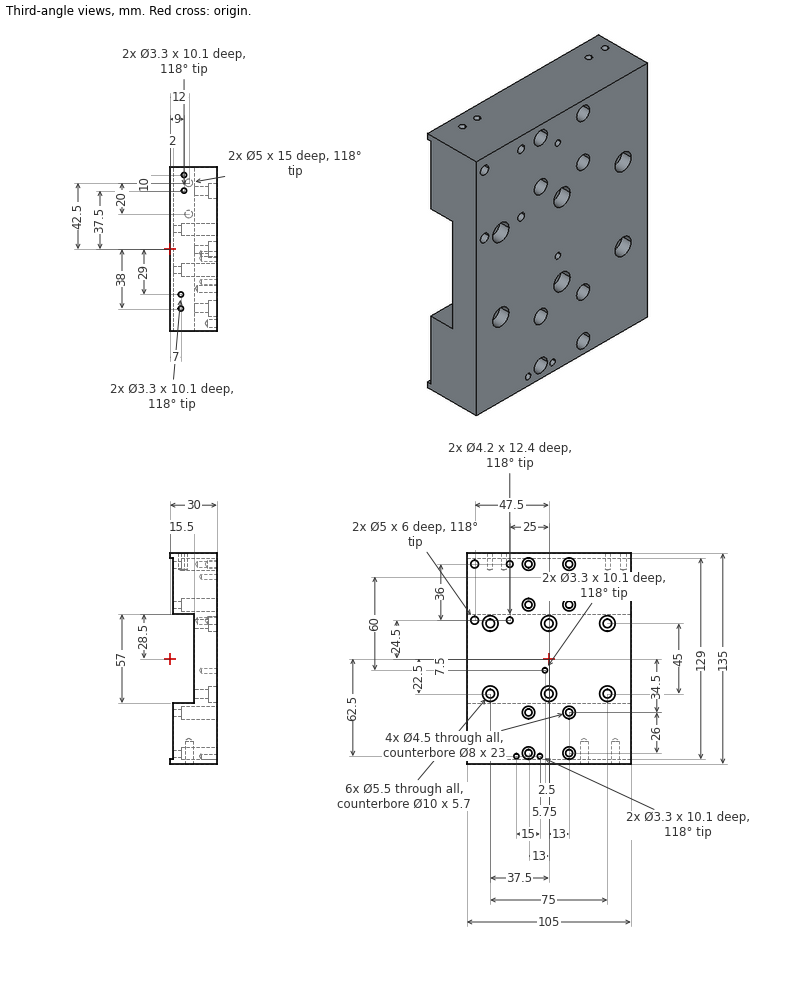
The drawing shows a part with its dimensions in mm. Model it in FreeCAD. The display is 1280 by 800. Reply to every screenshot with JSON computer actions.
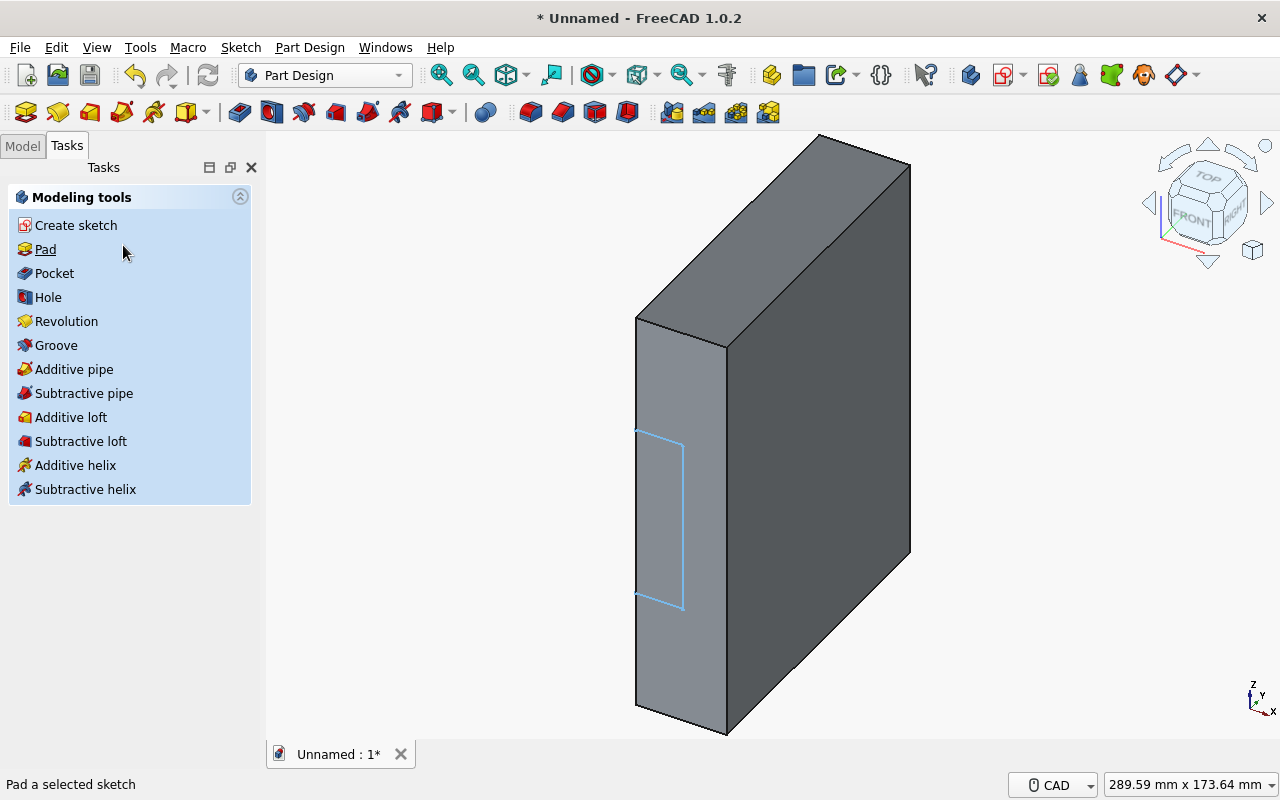
{"action": "left_click", "coordinate": [240, 112]}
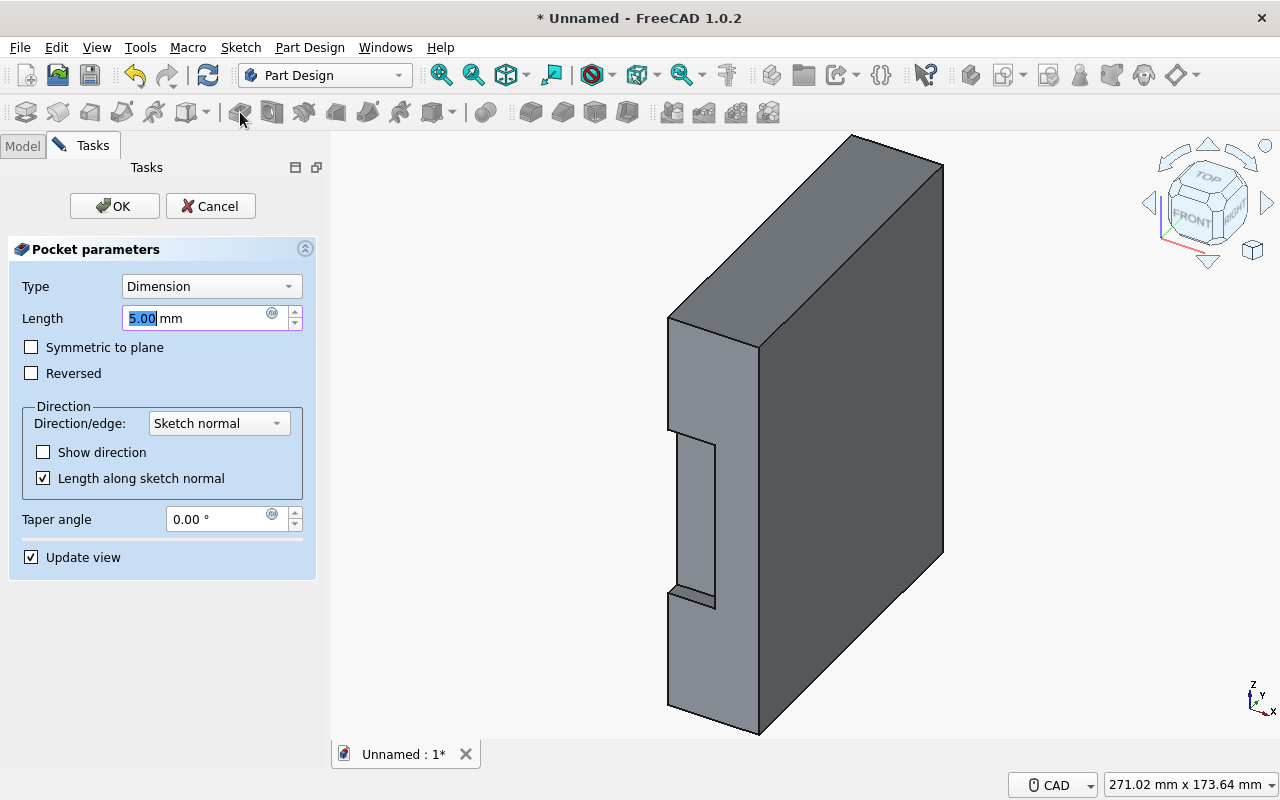
{"action": "left_click", "coordinate": [212, 286]}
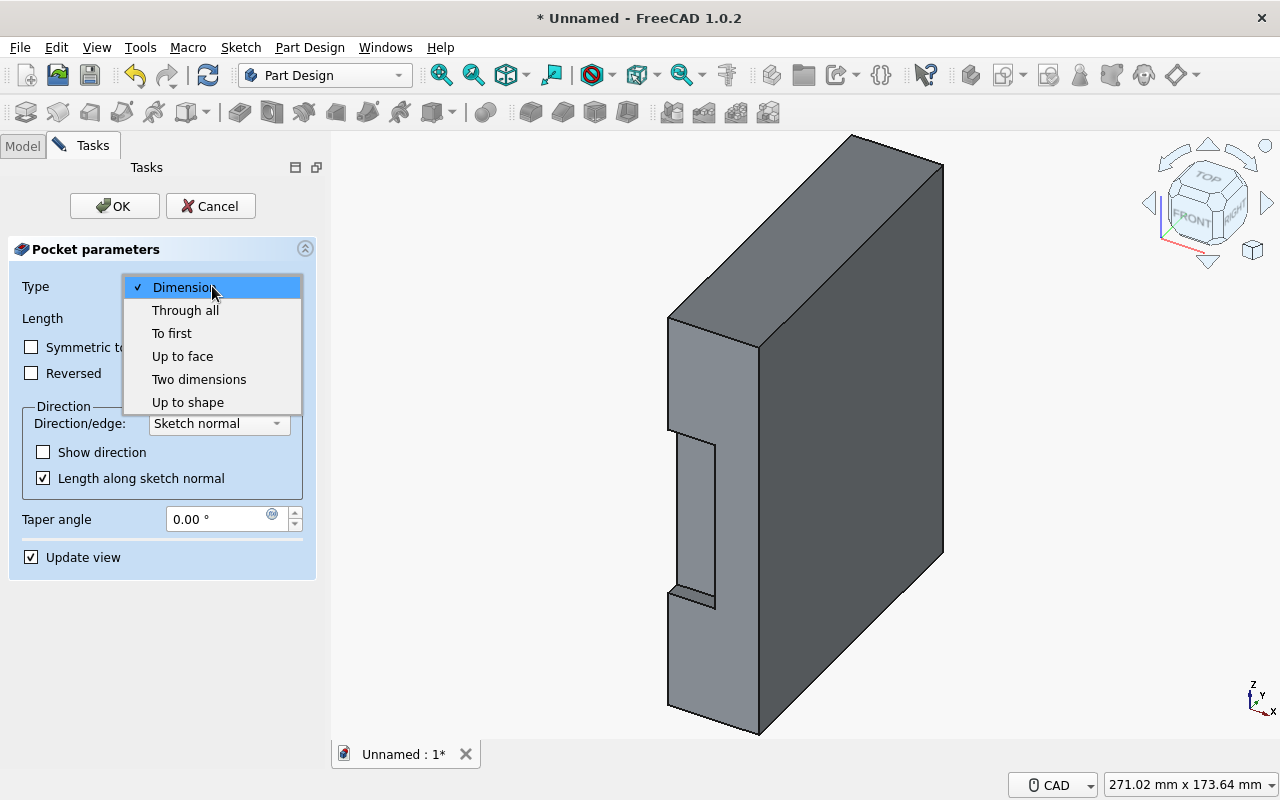
{"action": "left_click", "coordinate": [212, 310]}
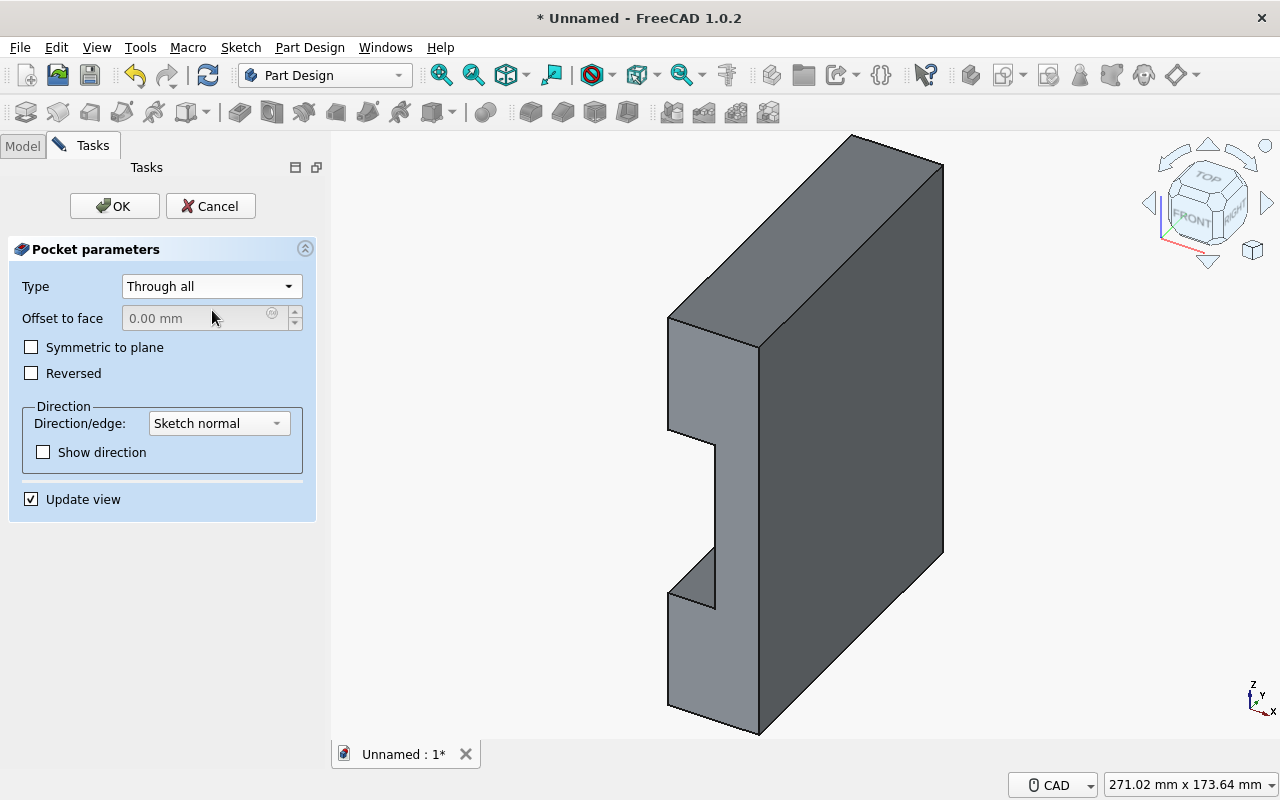
{"action": "left_click", "coordinate": [115, 206]}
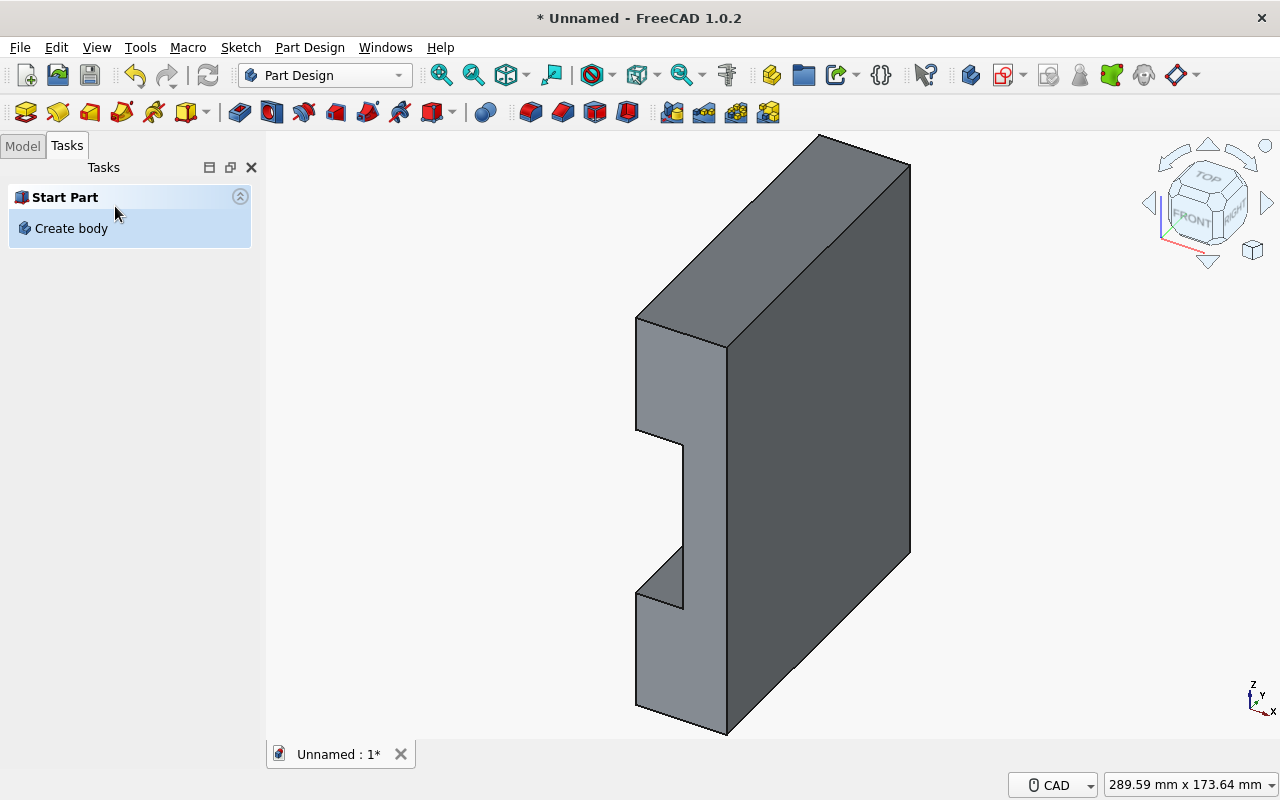
{"action": "left_click", "coordinate": [1004, 76]}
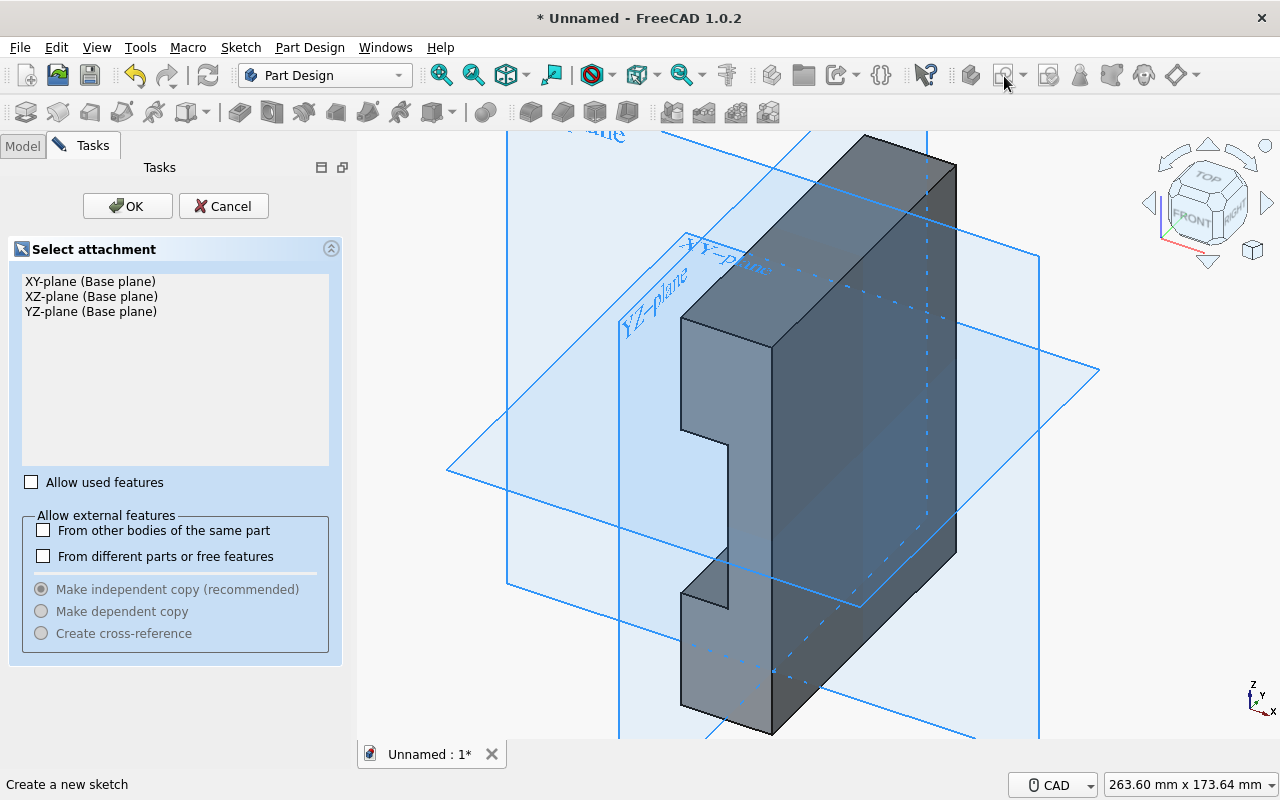
{"action": "left_click", "coordinate": [82, 312]}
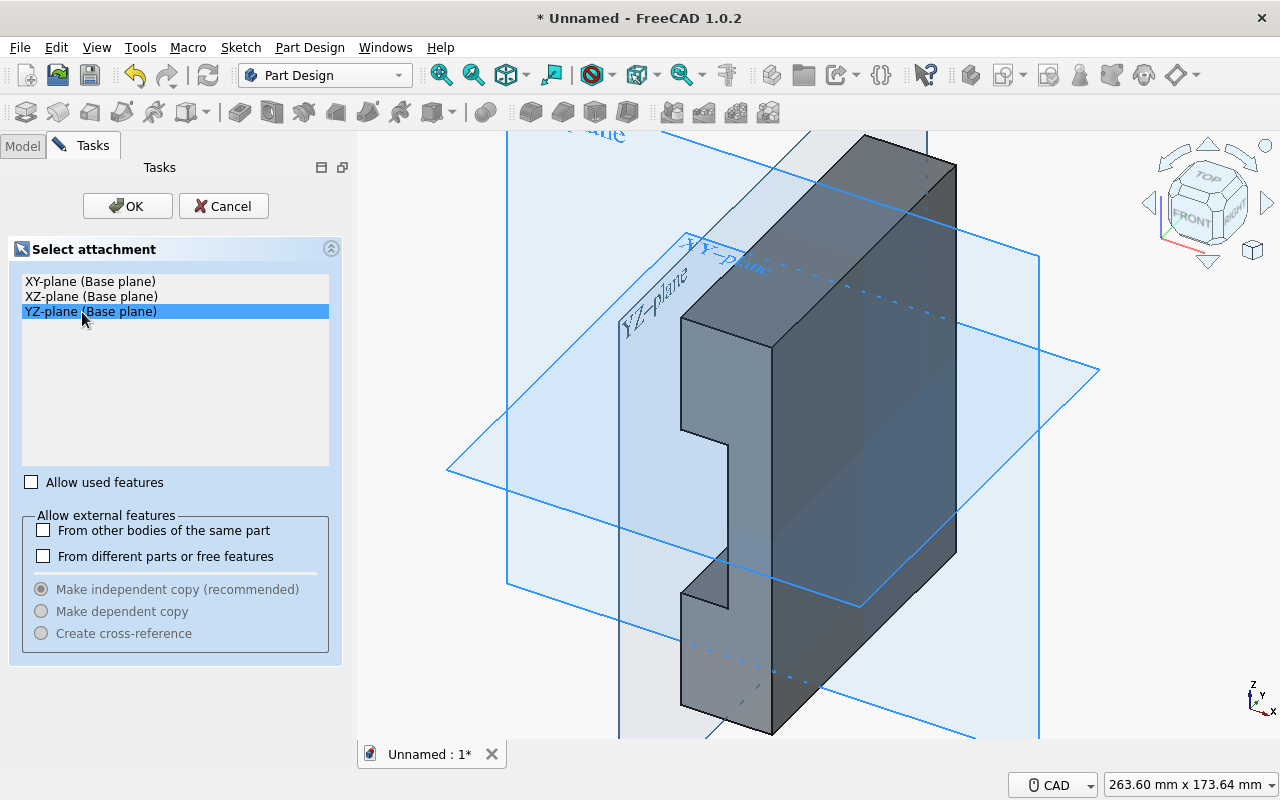
{"action": "left_click", "coordinate": [128, 206]}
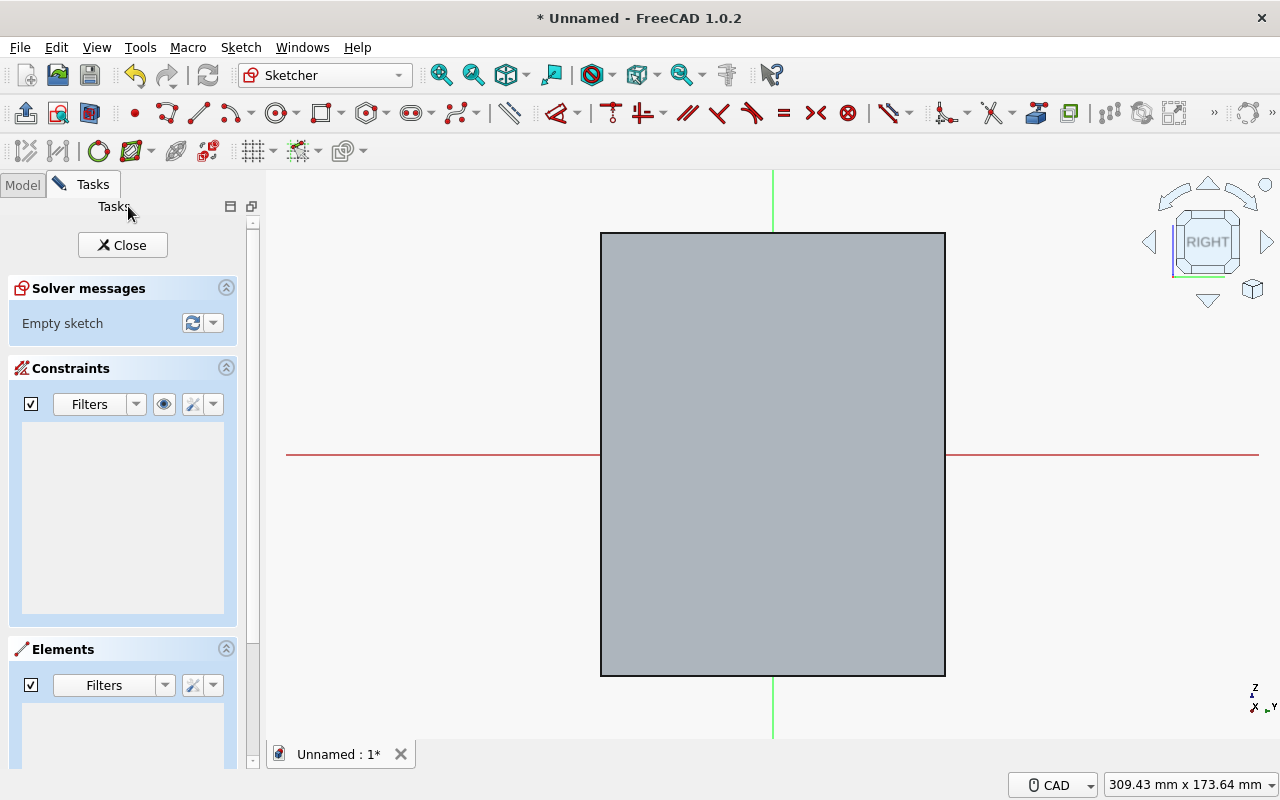
{"action": "left_click", "coordinate": [90, 114]}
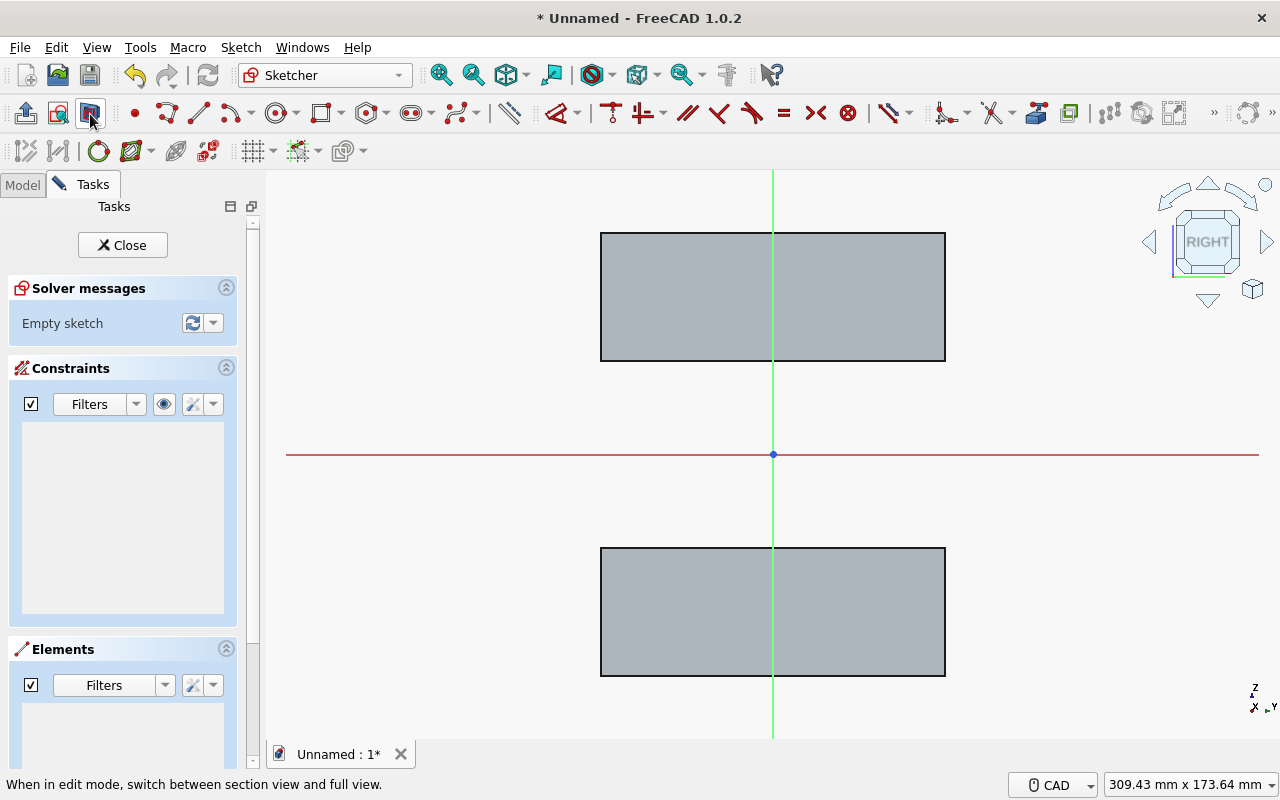
{"action": "left_click", "coordinate": [344, 114]}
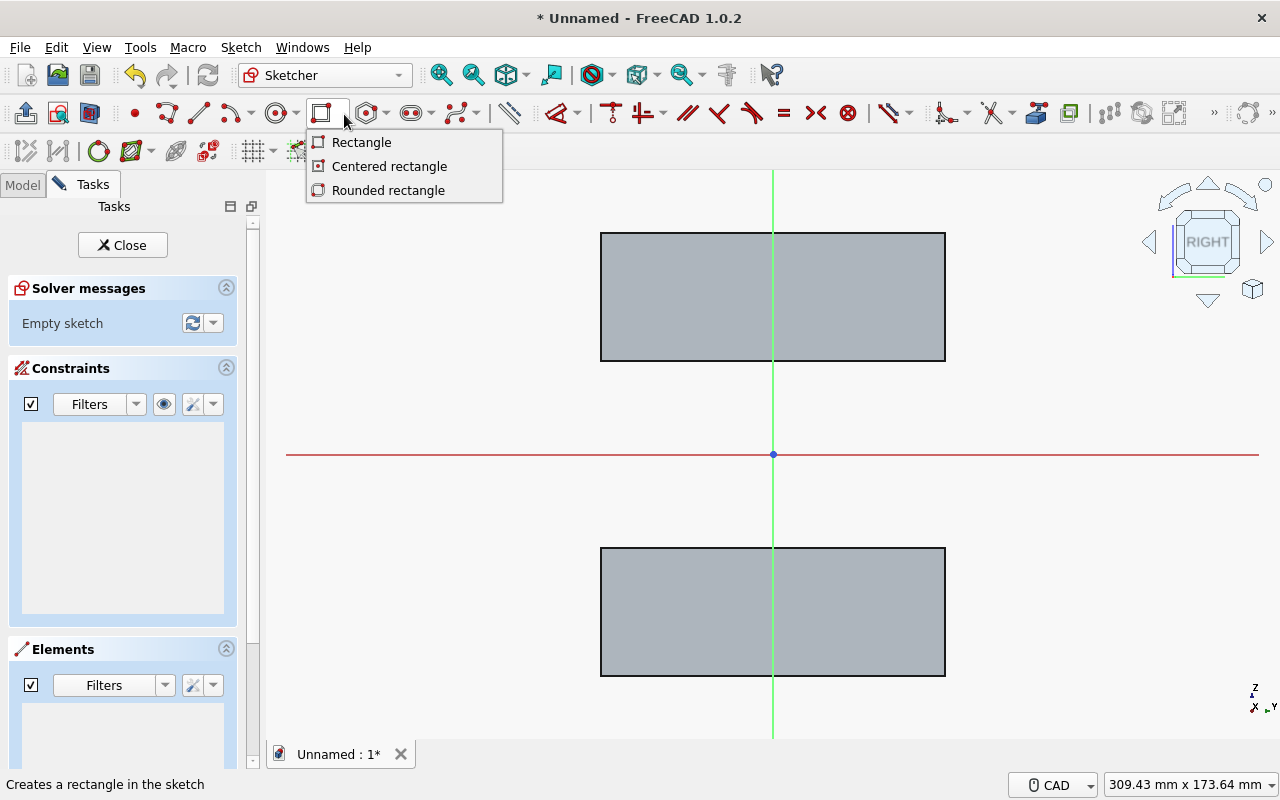
{"action": "left_click", "coordinate": [404, 166]}